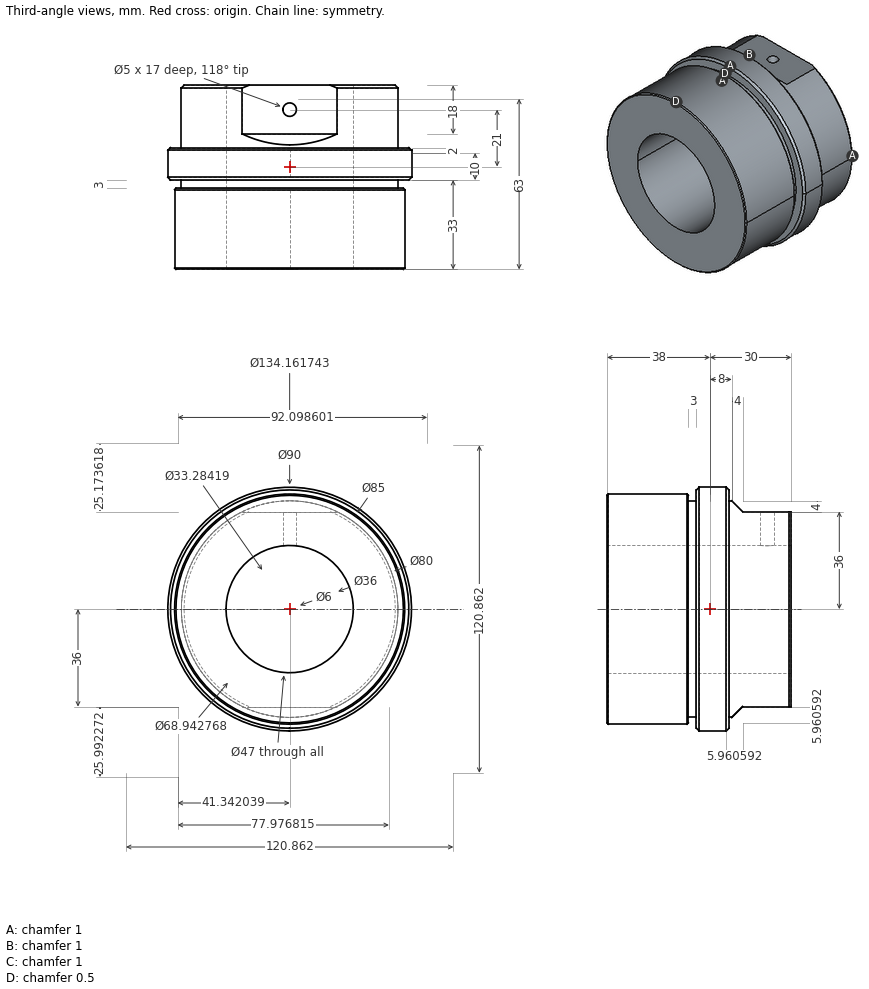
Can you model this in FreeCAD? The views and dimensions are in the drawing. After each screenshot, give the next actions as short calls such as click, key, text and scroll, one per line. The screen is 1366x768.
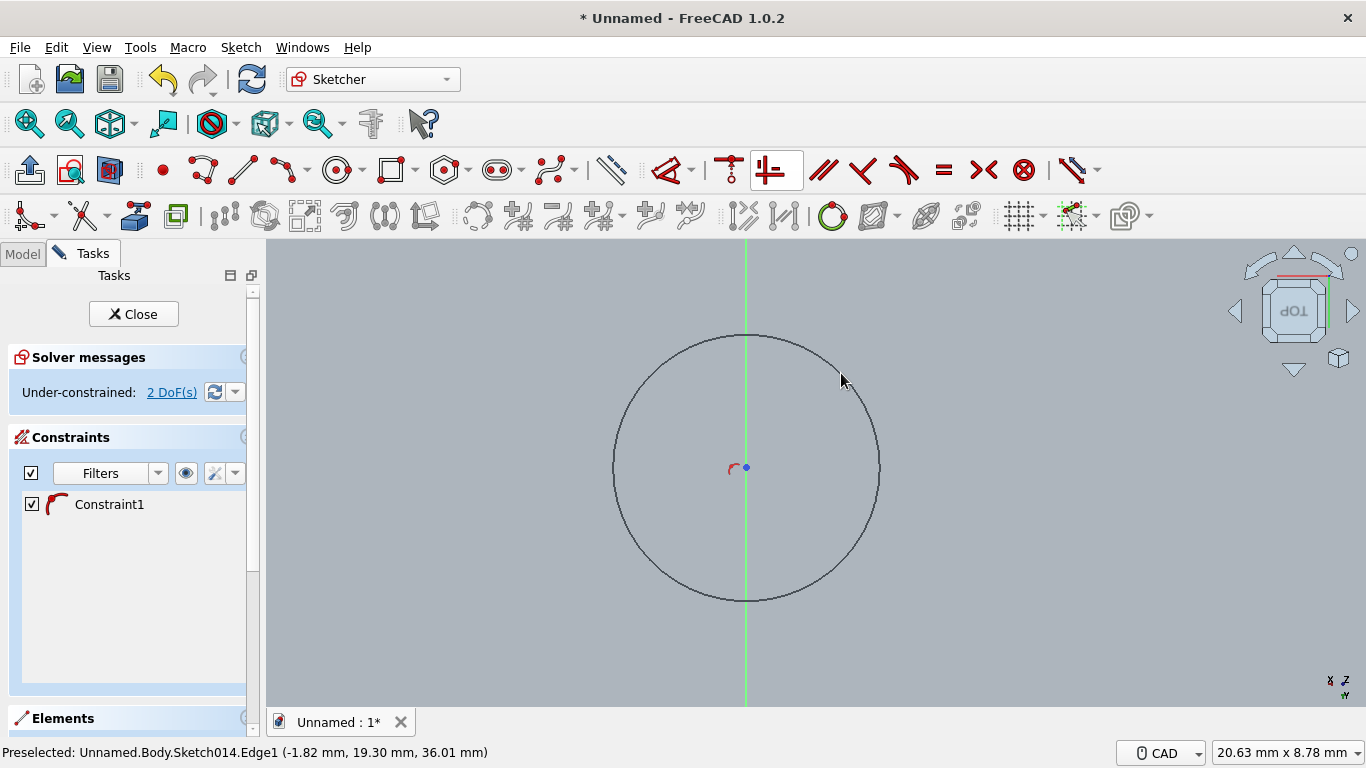
click(666, 170)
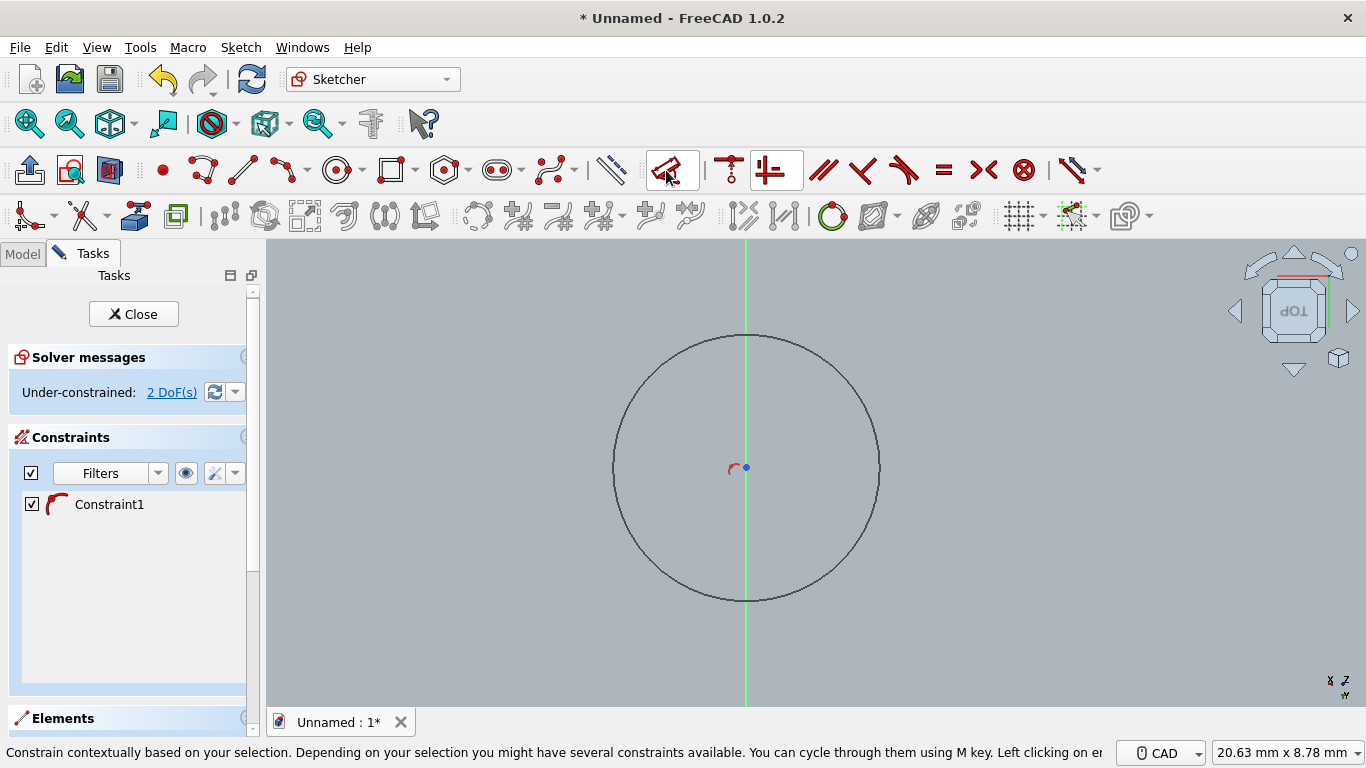
click(840, 373)
click(862, 350)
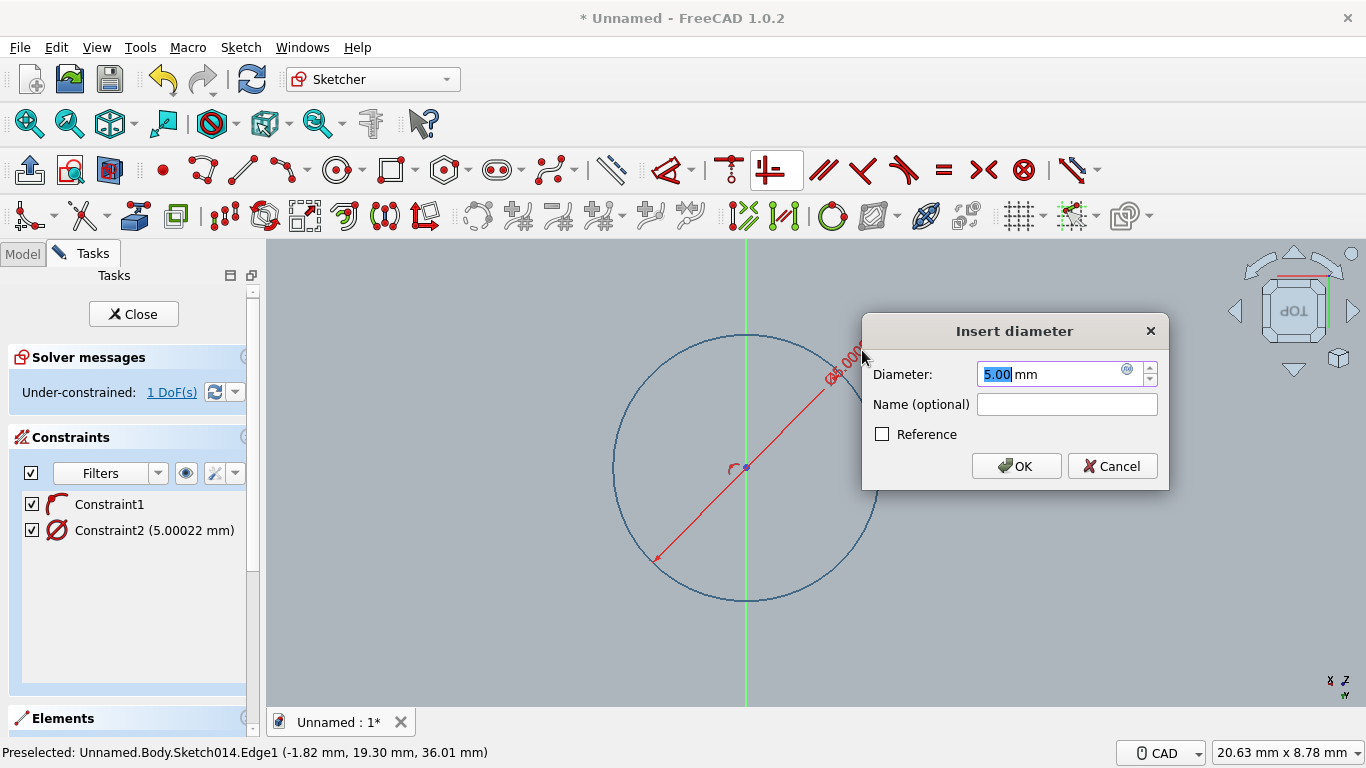
text(5)
key(Return)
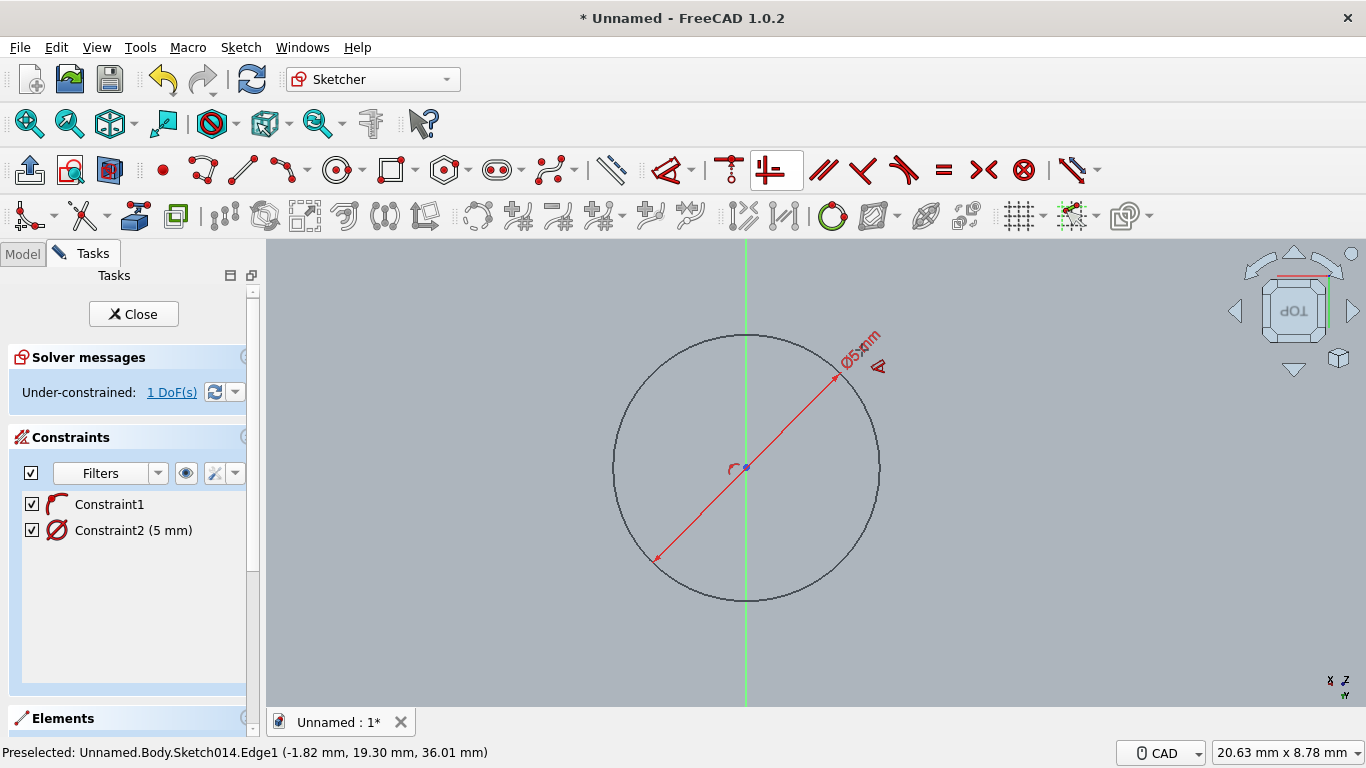
click(746, 468)
click(780, 368)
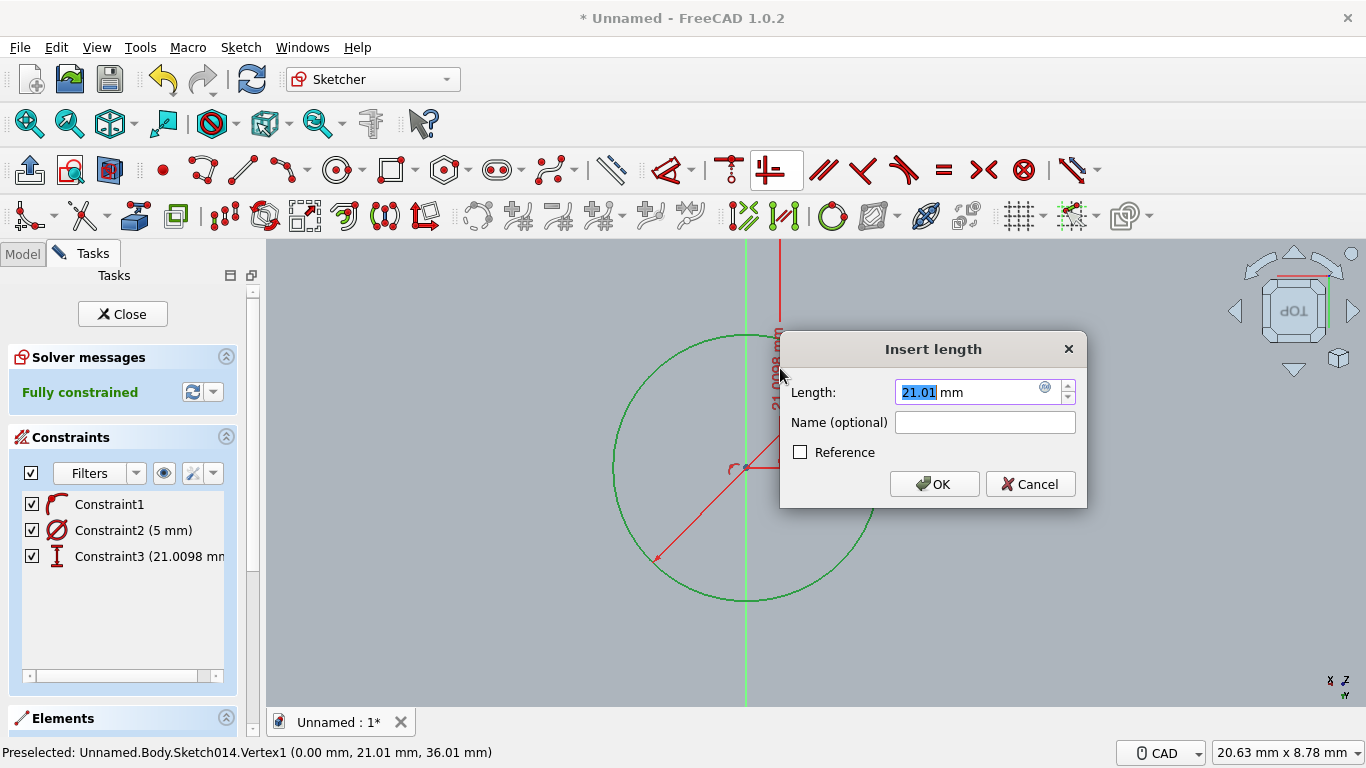
text(21)
key(Return)
key(Escape)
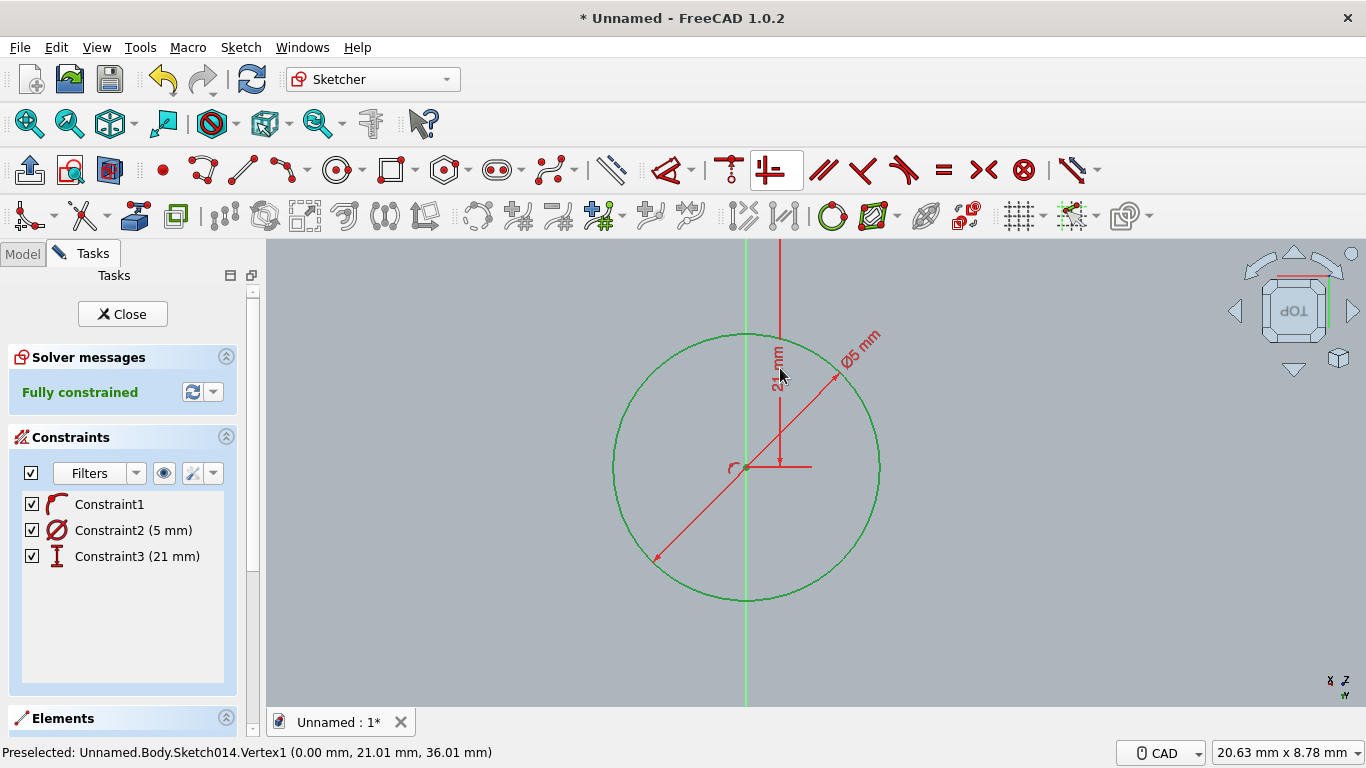
click(123, 314)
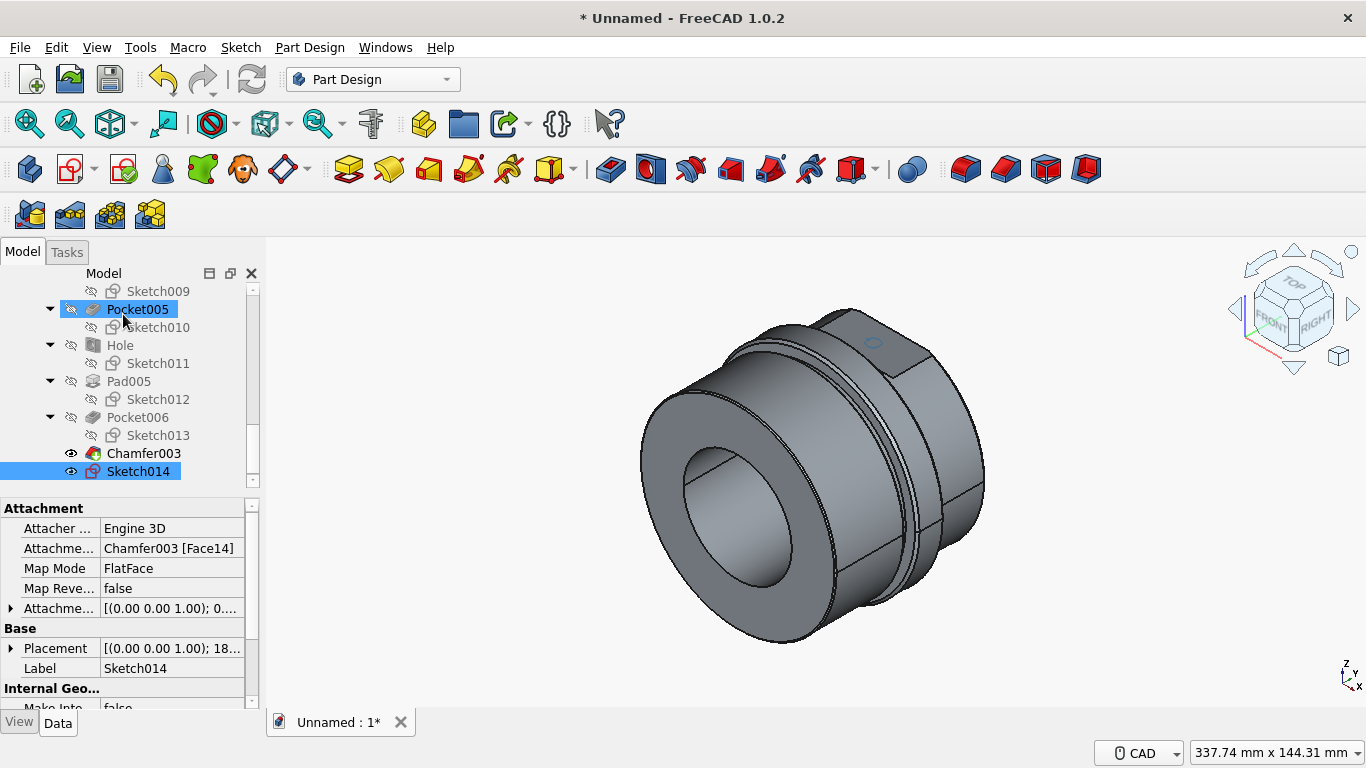
click(652, 170)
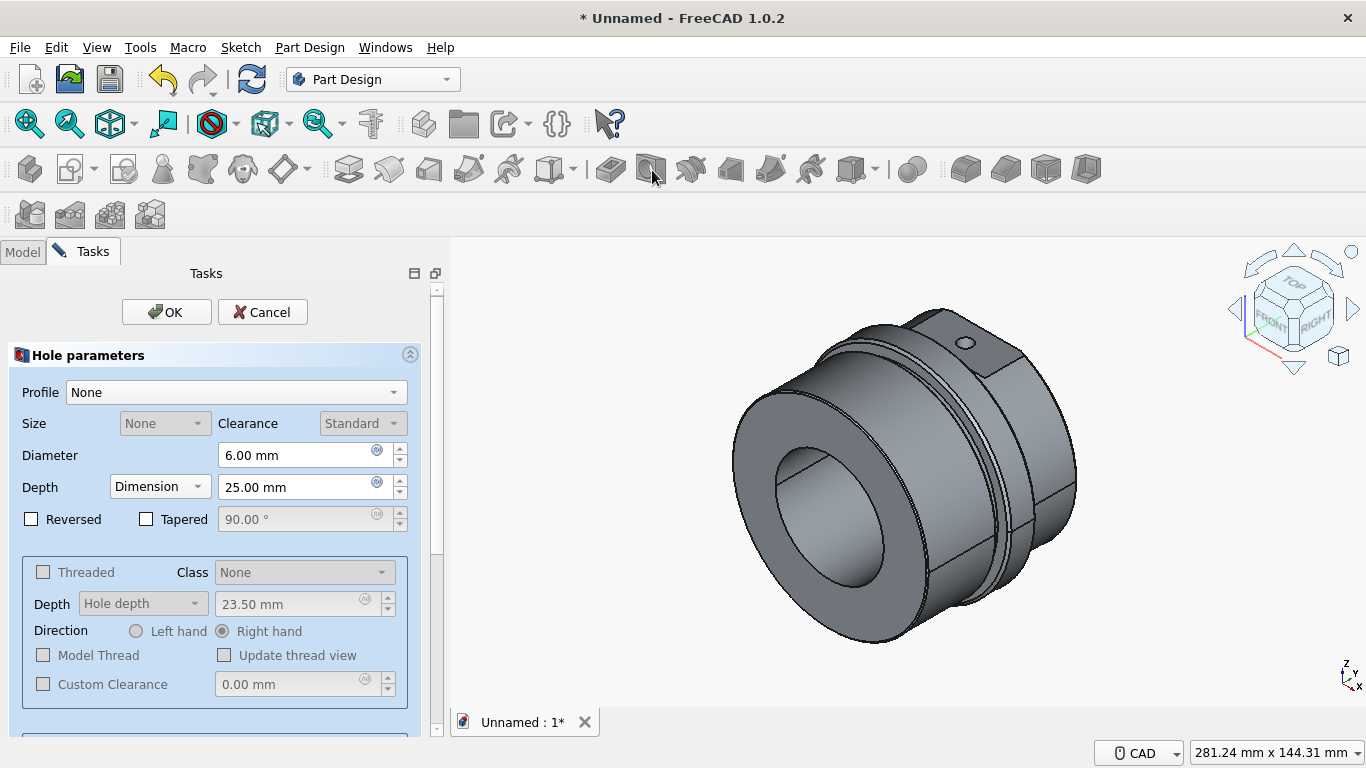
triple_click(305, 455)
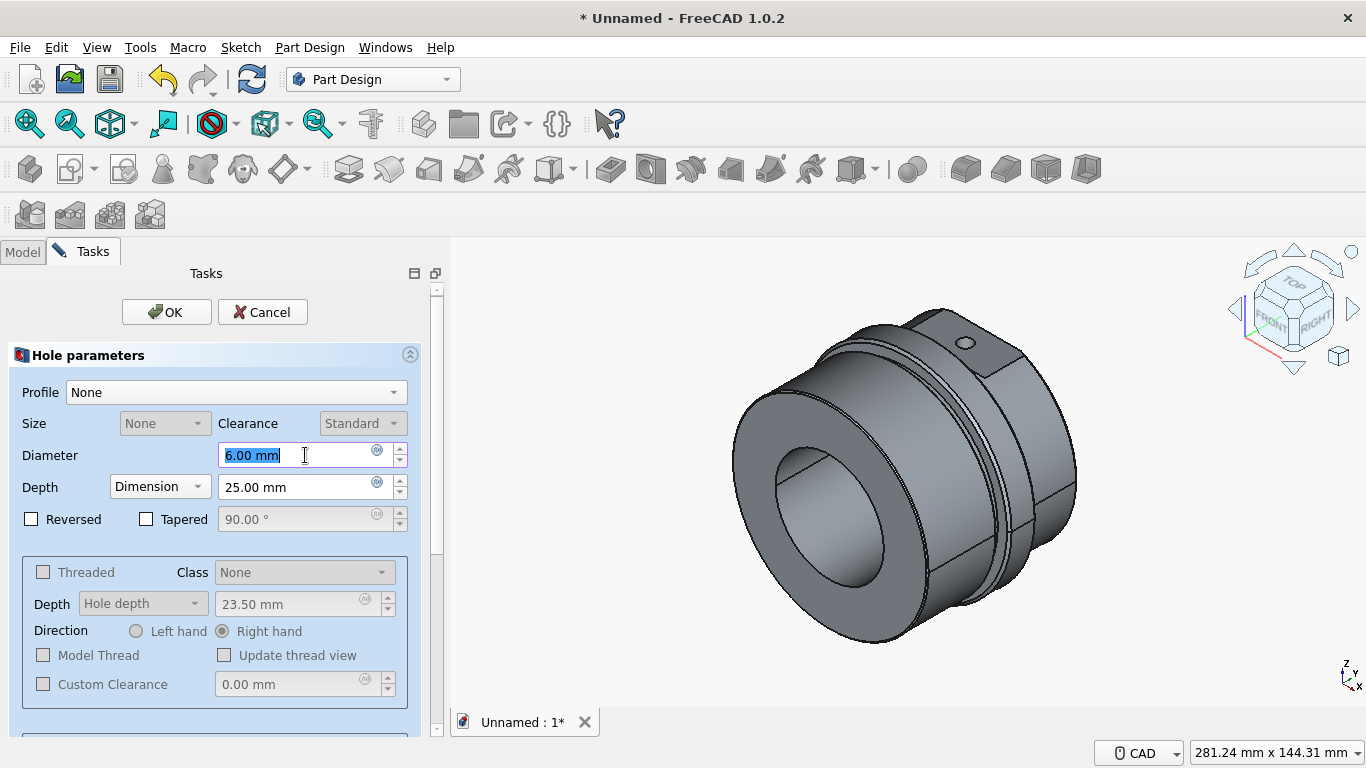
text(5)
key(Tab)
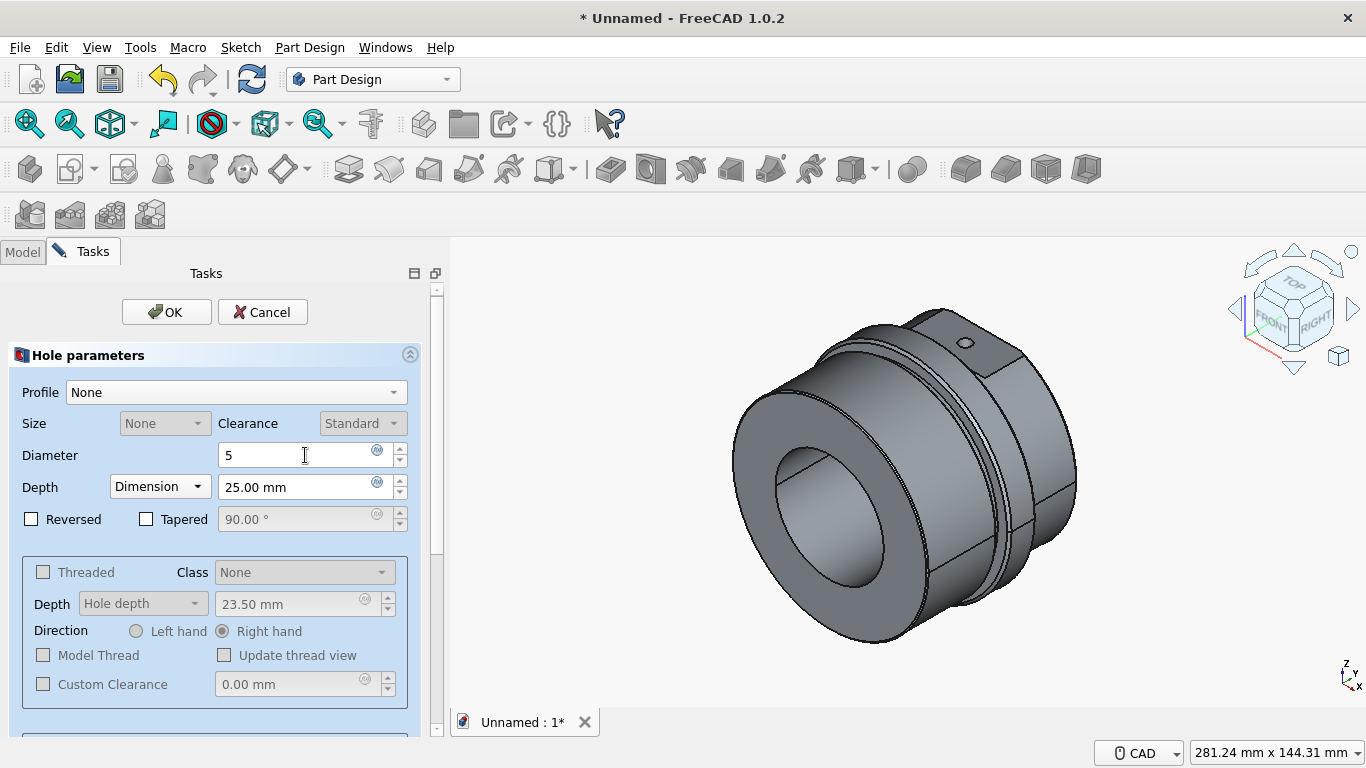
triple_click(305, 487)